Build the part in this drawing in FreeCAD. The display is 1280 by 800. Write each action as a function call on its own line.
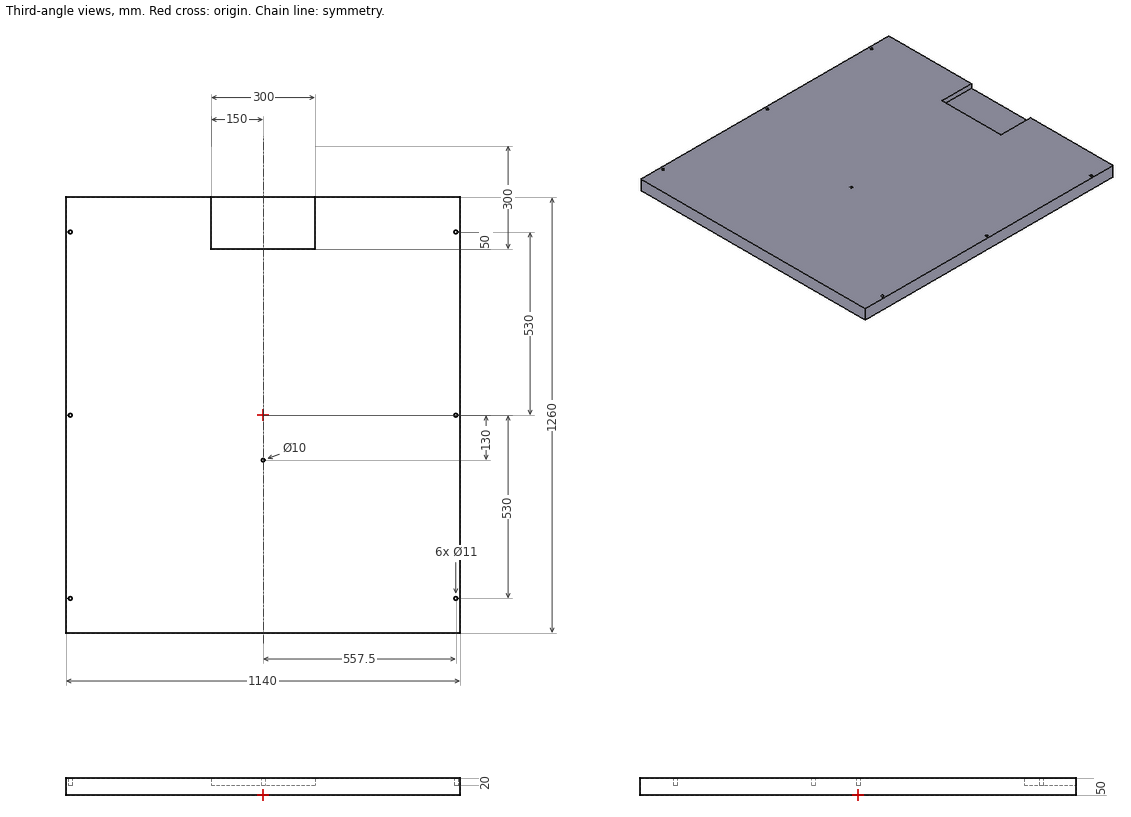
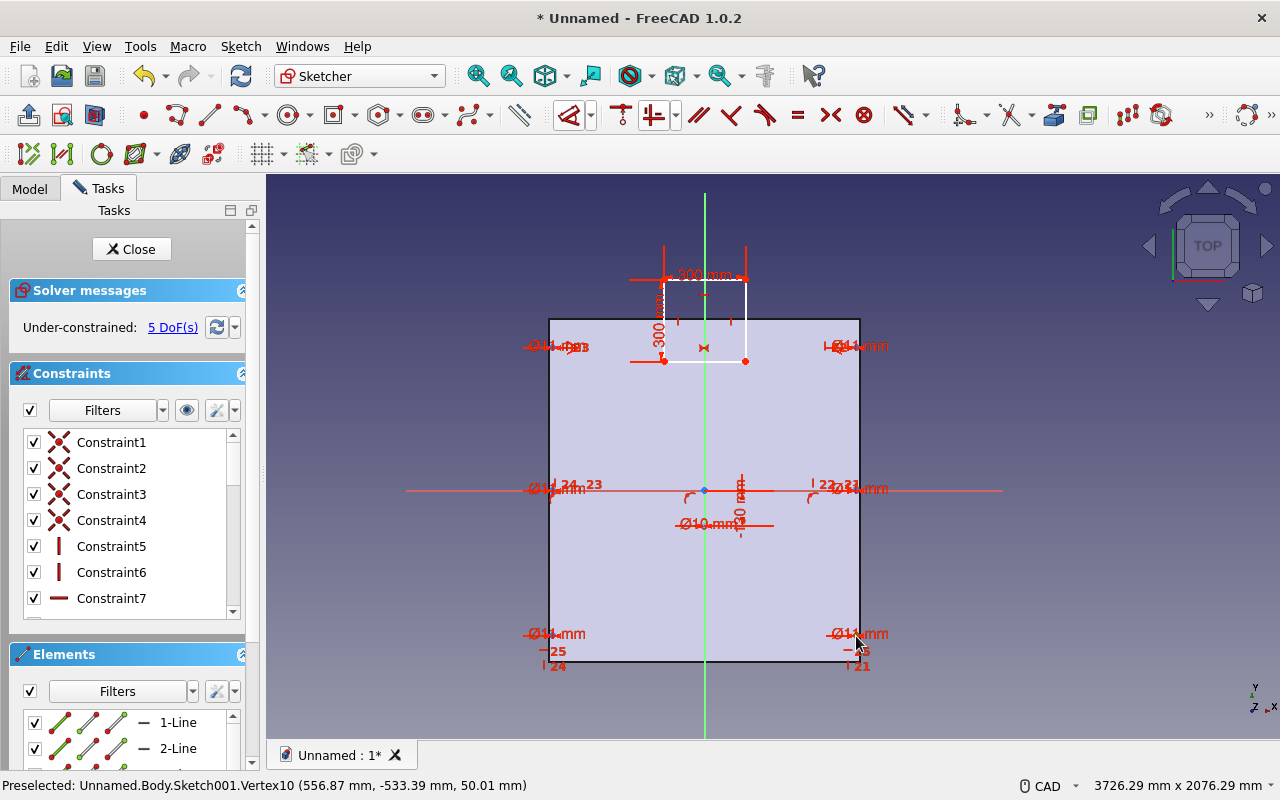
key(i)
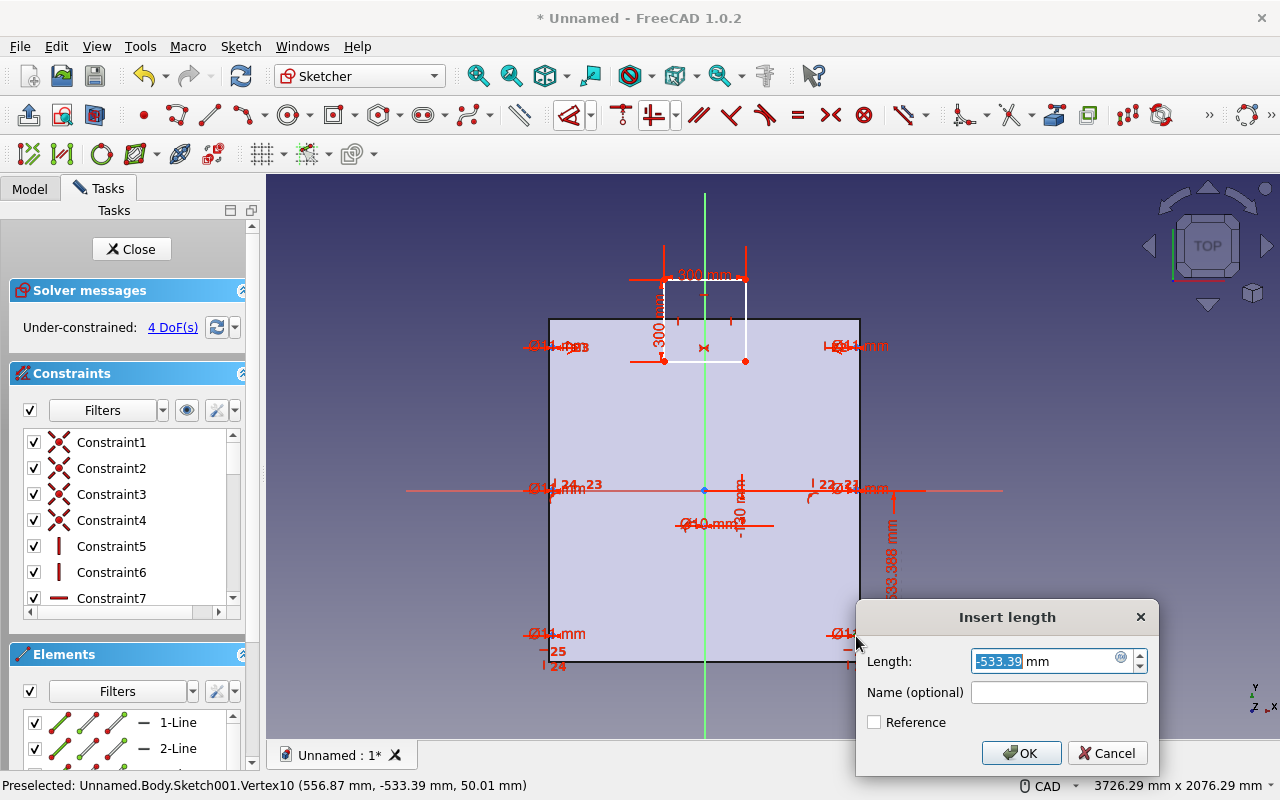
text(-530)
key(Return)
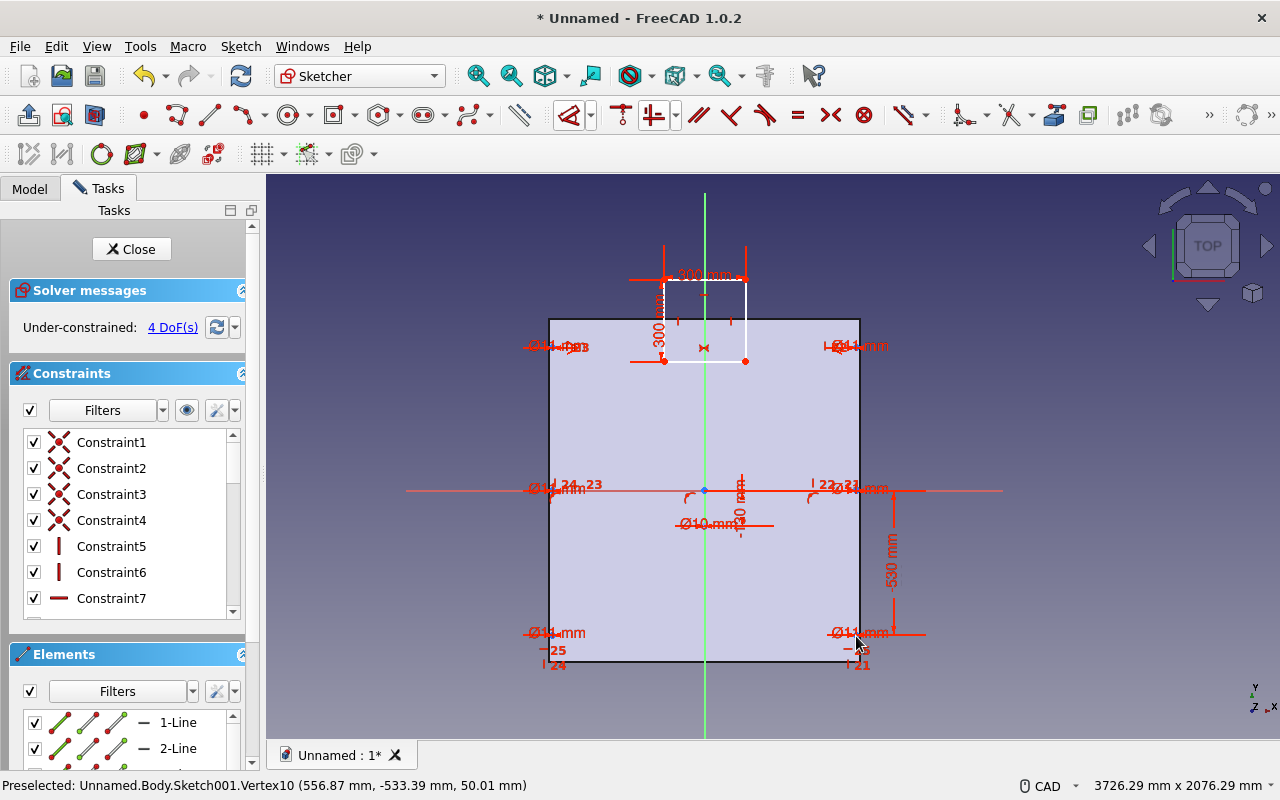
click(856, 348)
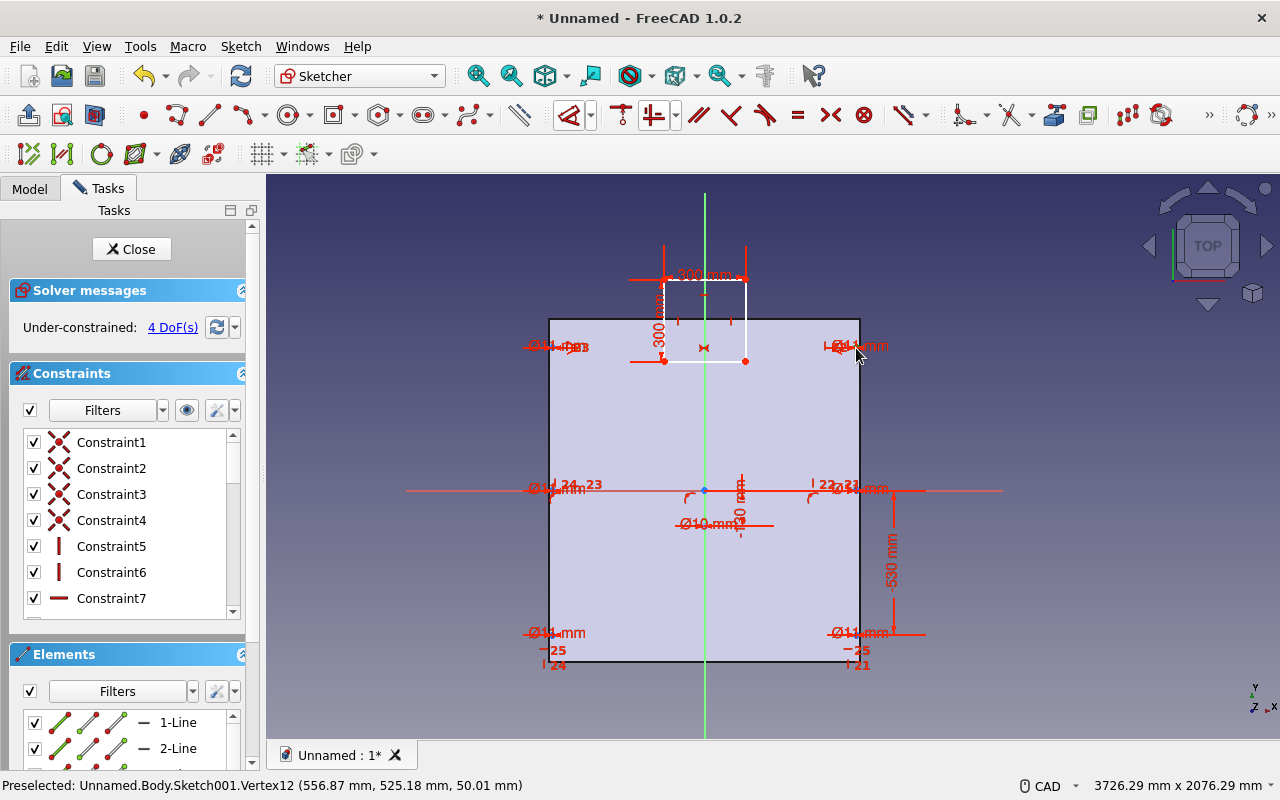
key(i)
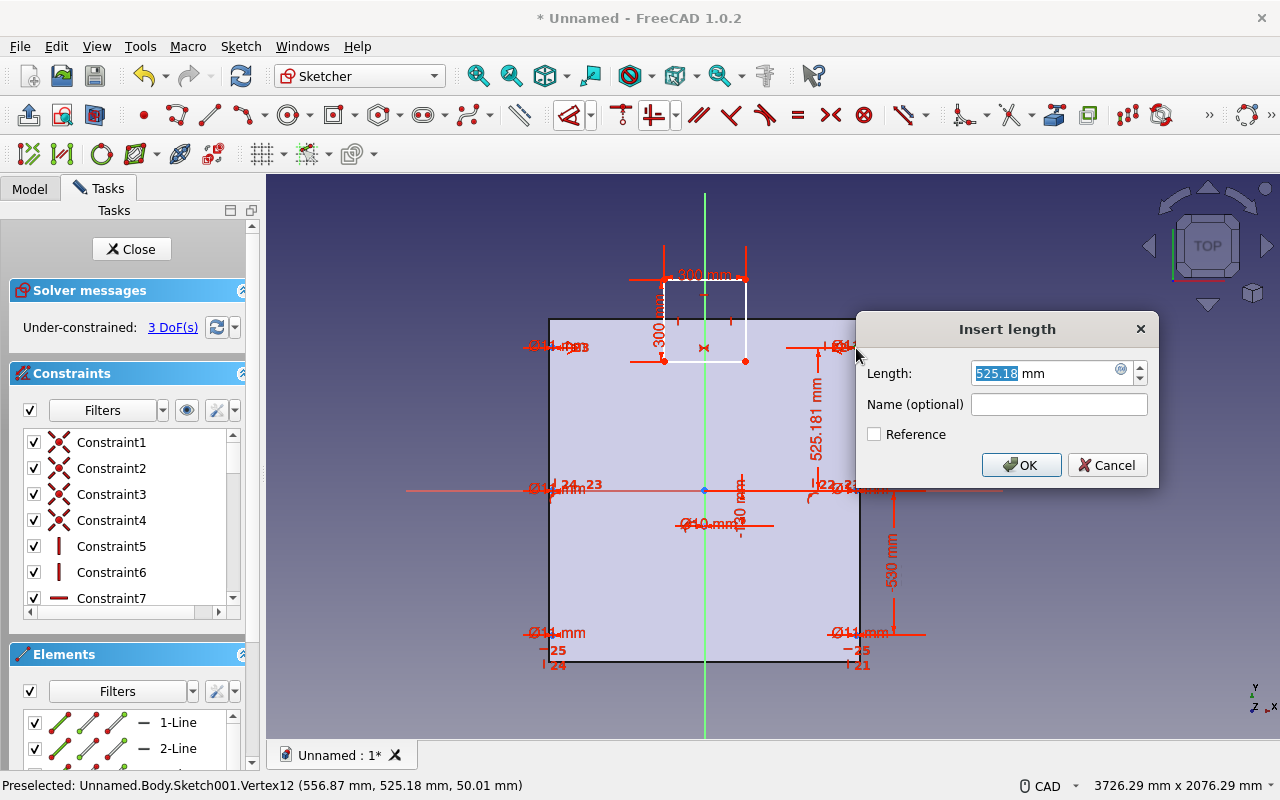
text(530)
key(Return)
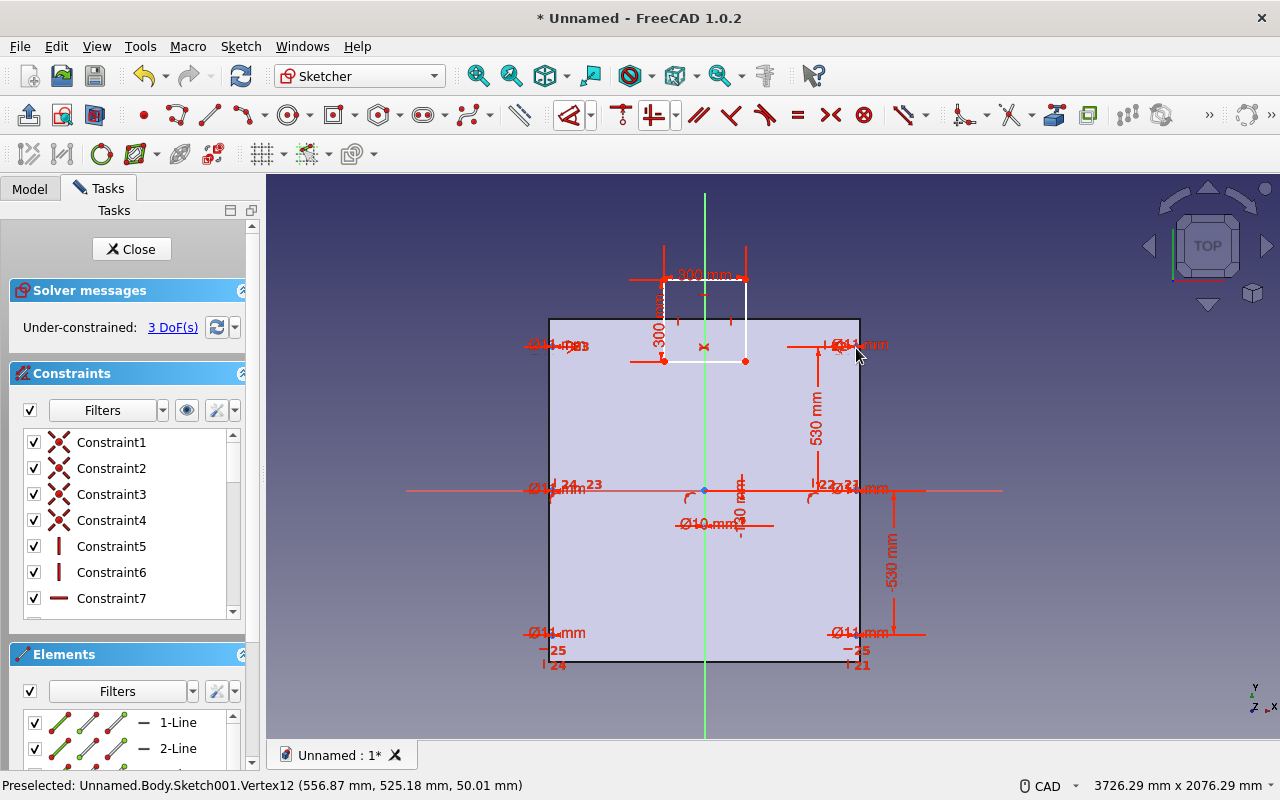
scroll(746, 362, up, 6)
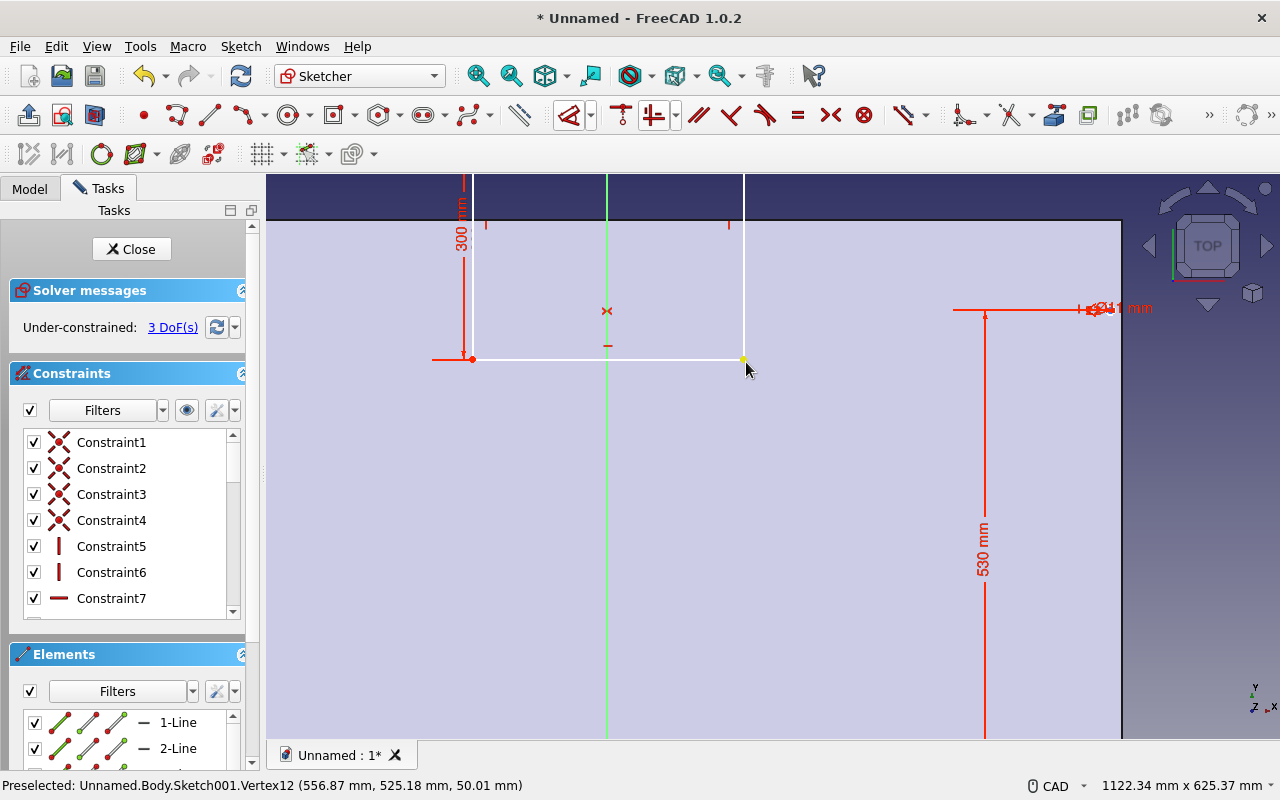
click(744, 360)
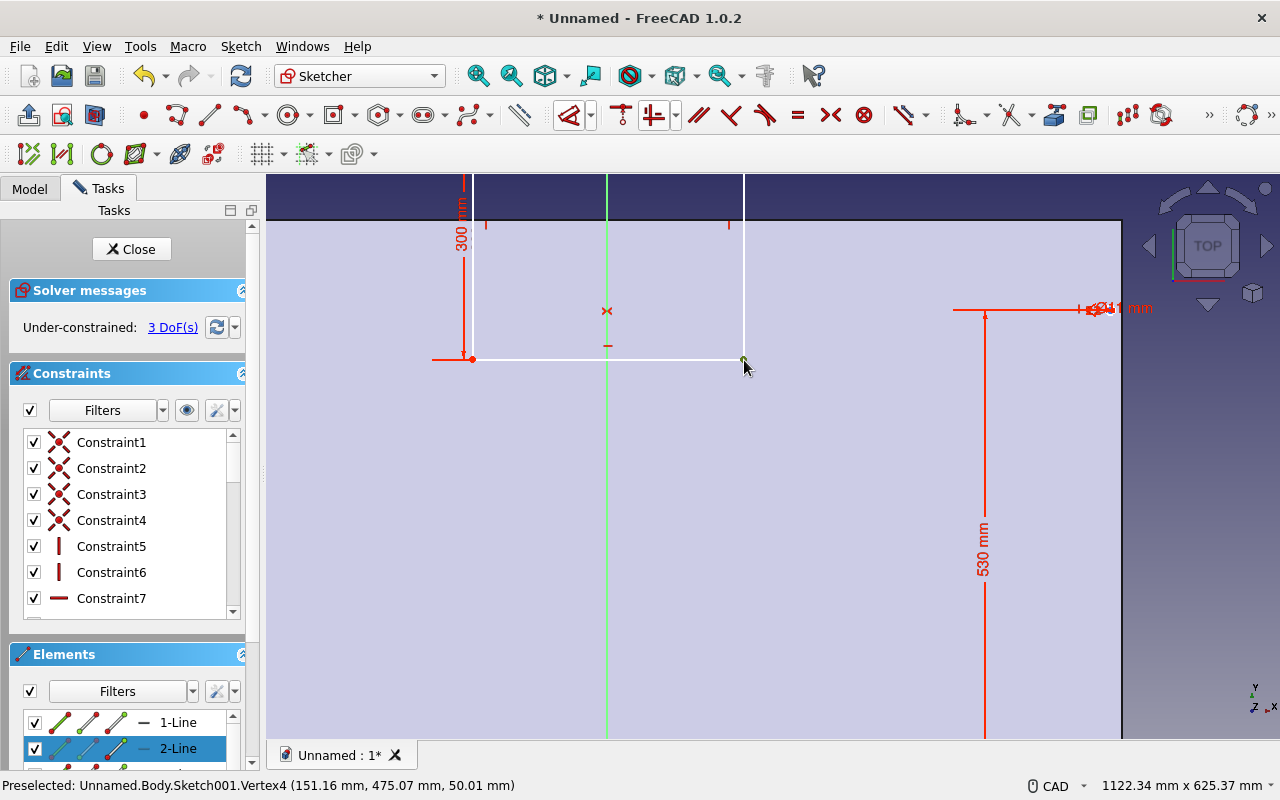
click(1110, 310)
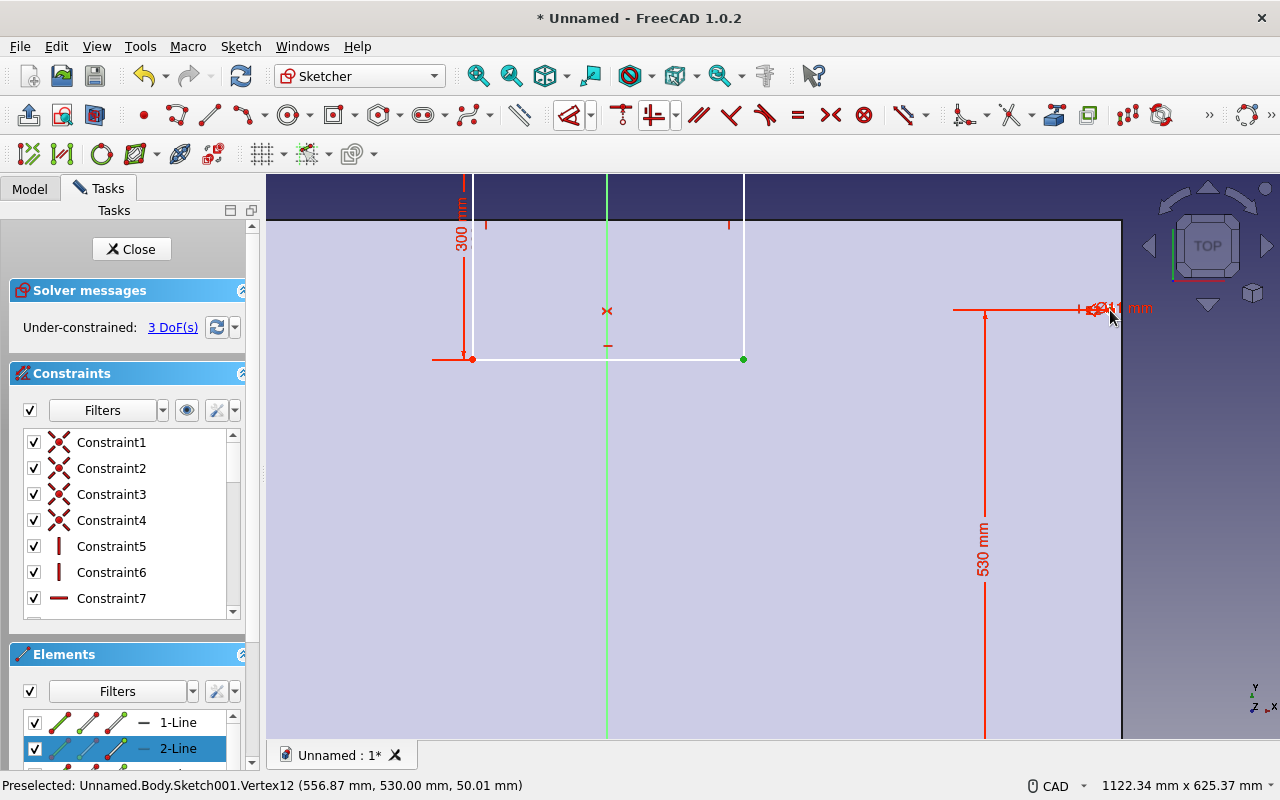
click(590, 116)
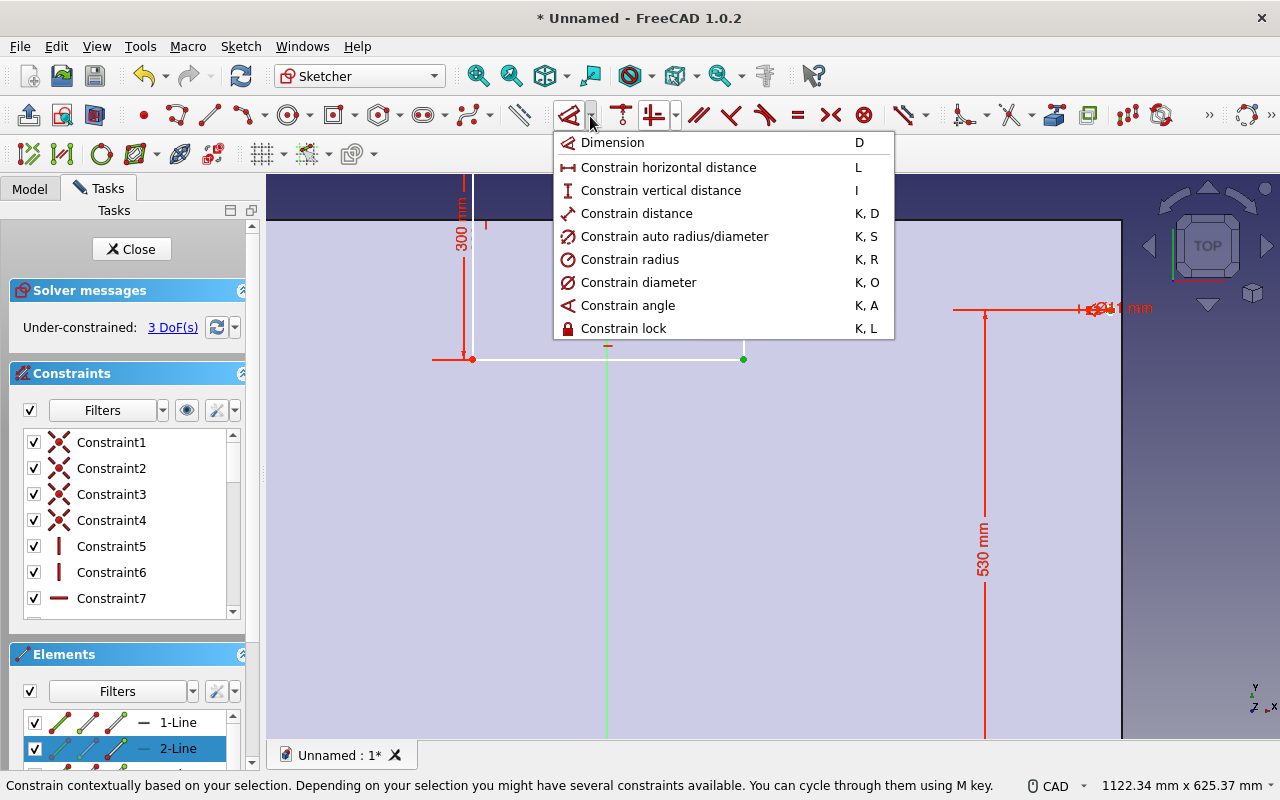
click(724, 190)